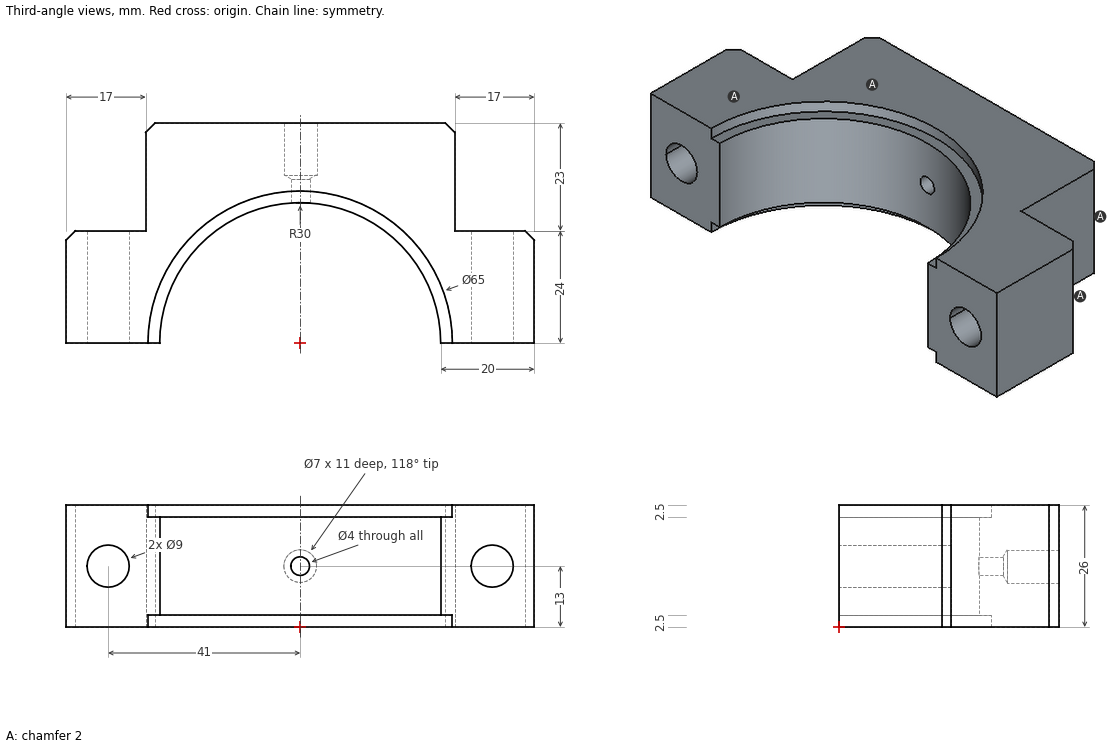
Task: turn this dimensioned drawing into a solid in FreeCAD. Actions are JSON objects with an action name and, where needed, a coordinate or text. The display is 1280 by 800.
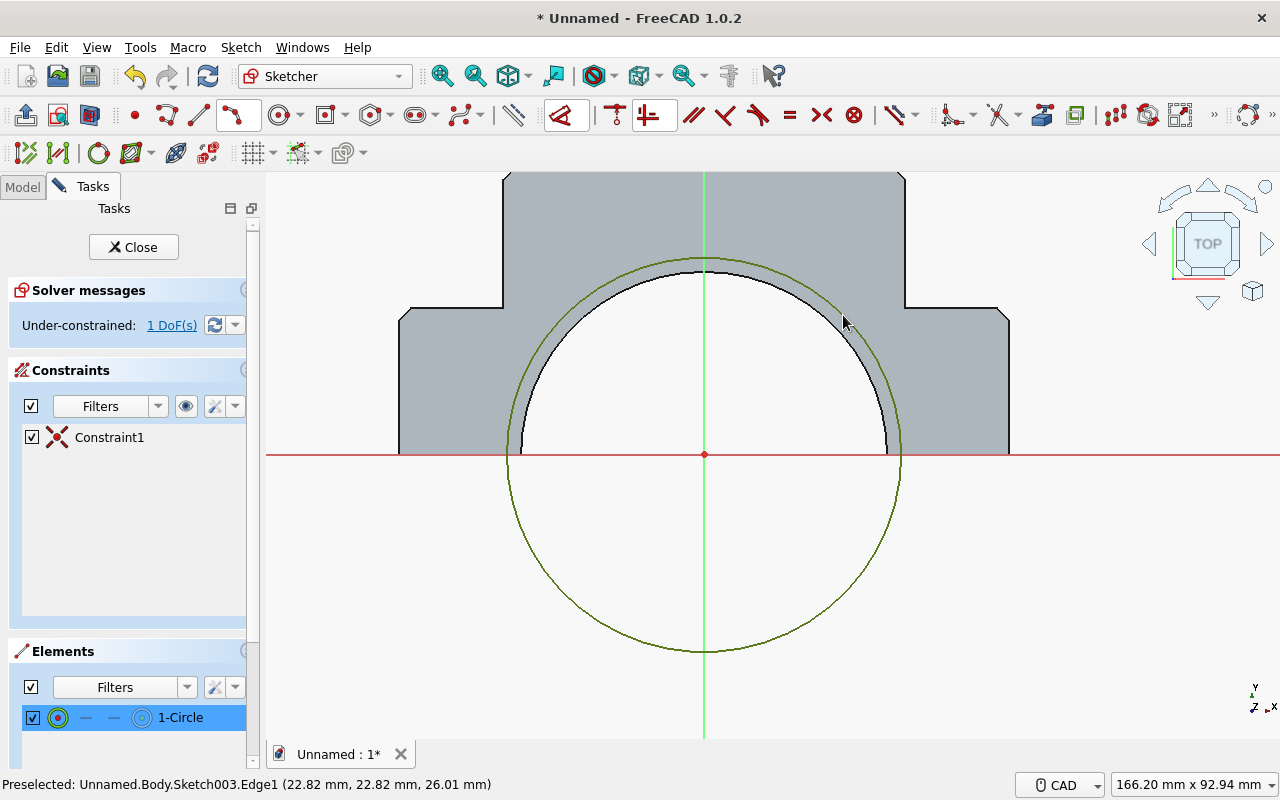
{"action": "key", "text": "k o"}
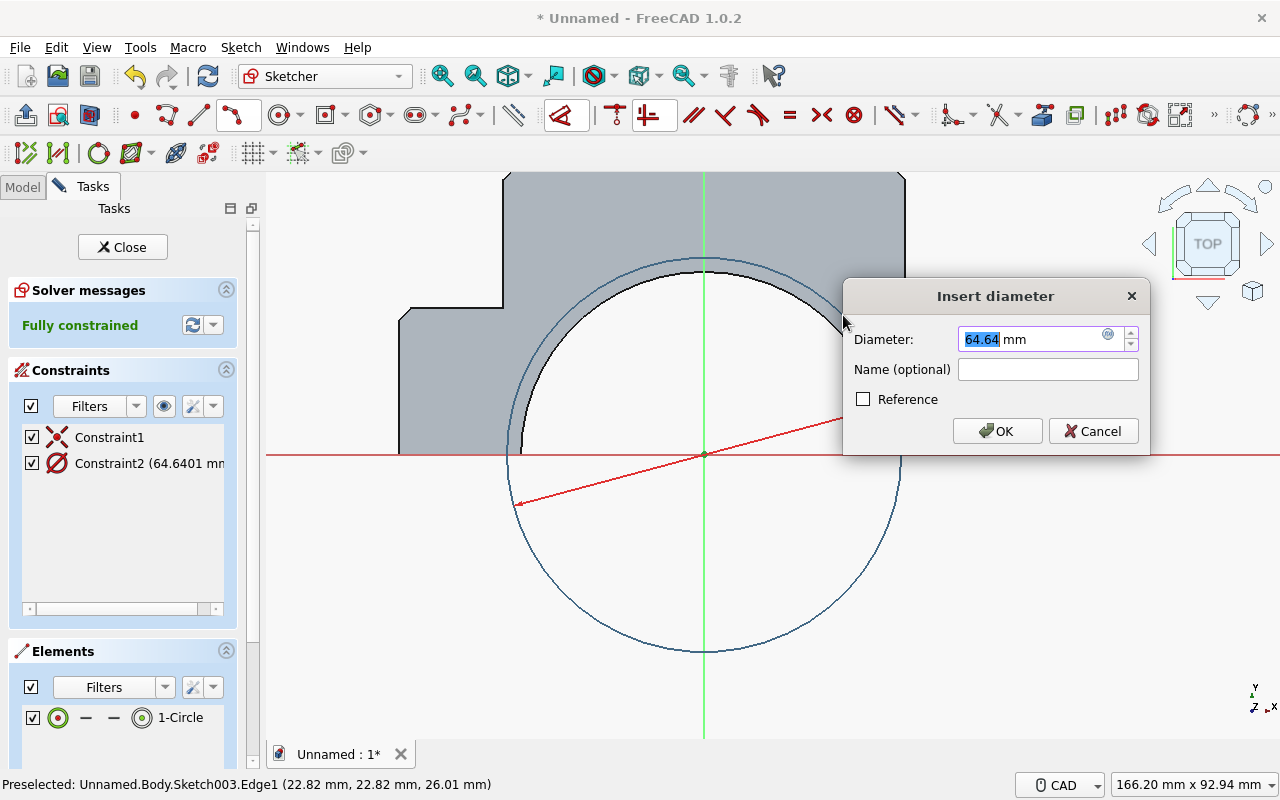
{"action": "type", "text": "65"}
{"action": "key", "text": "Return"}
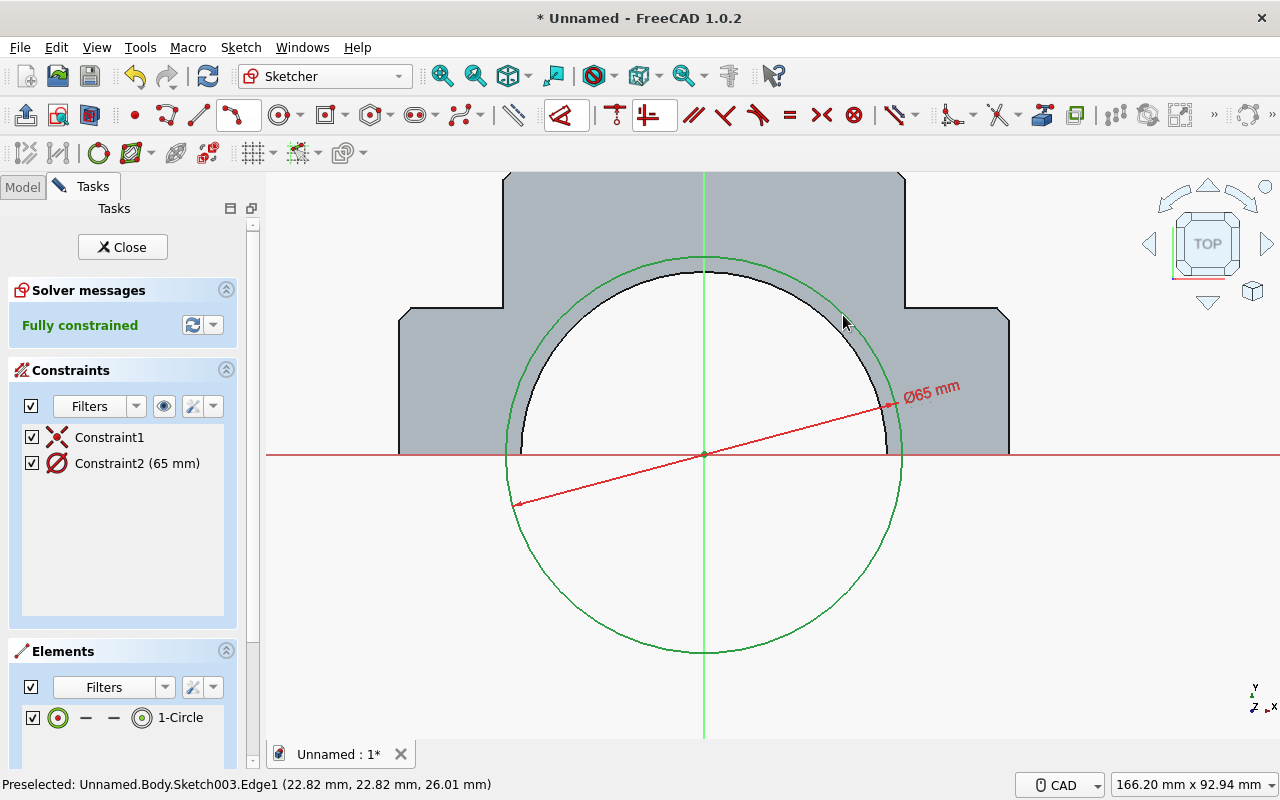
{"action": "left_click", "coordinate": [123, 247]}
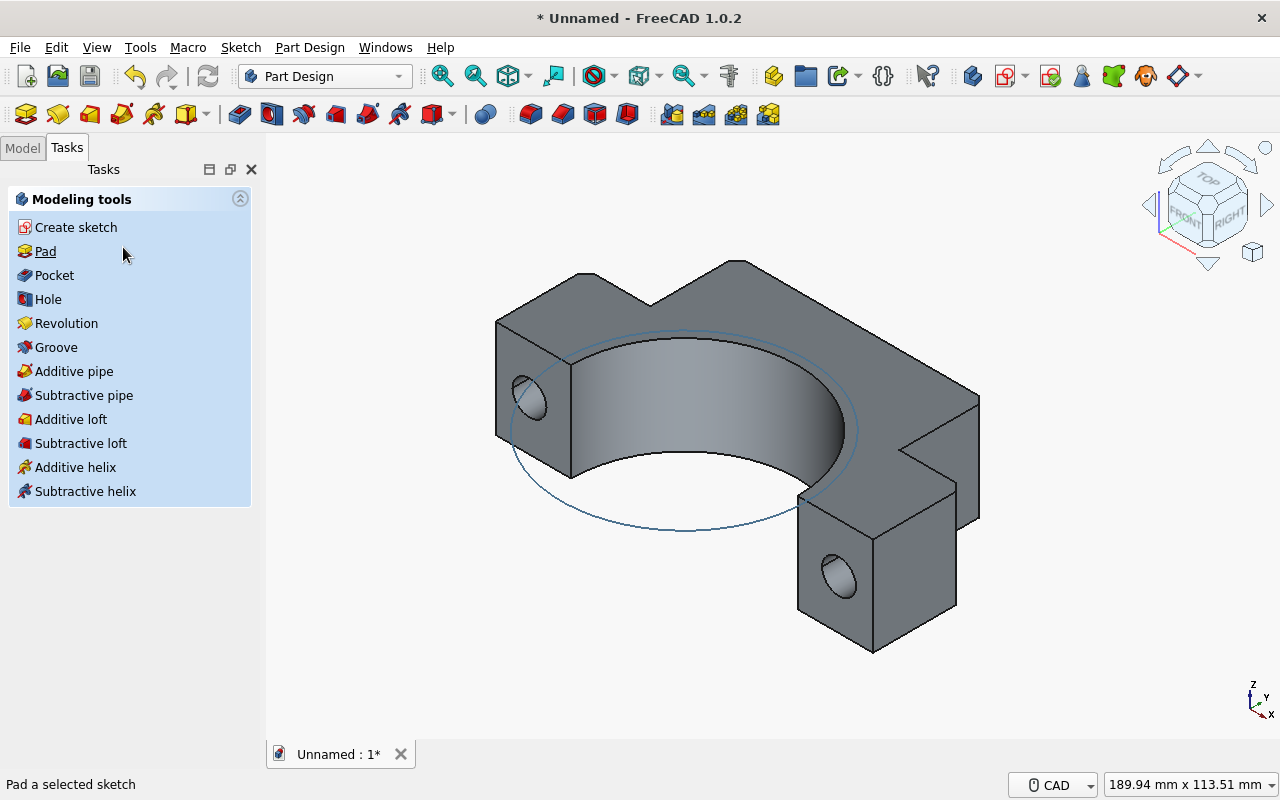
{"action": "left_click", "coordinate": [240, 114]}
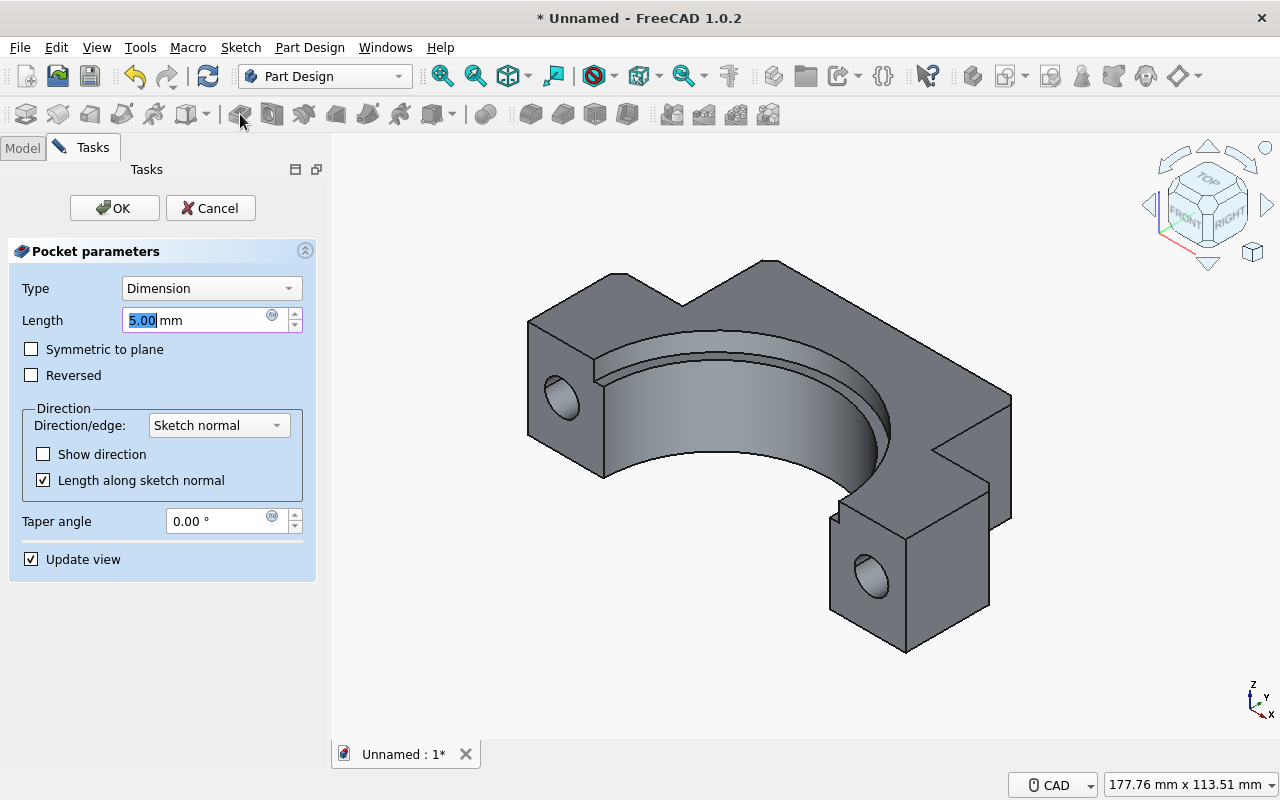
{"action": "type", "text": "2.5"}
{"action": "key", "text": "Tab"}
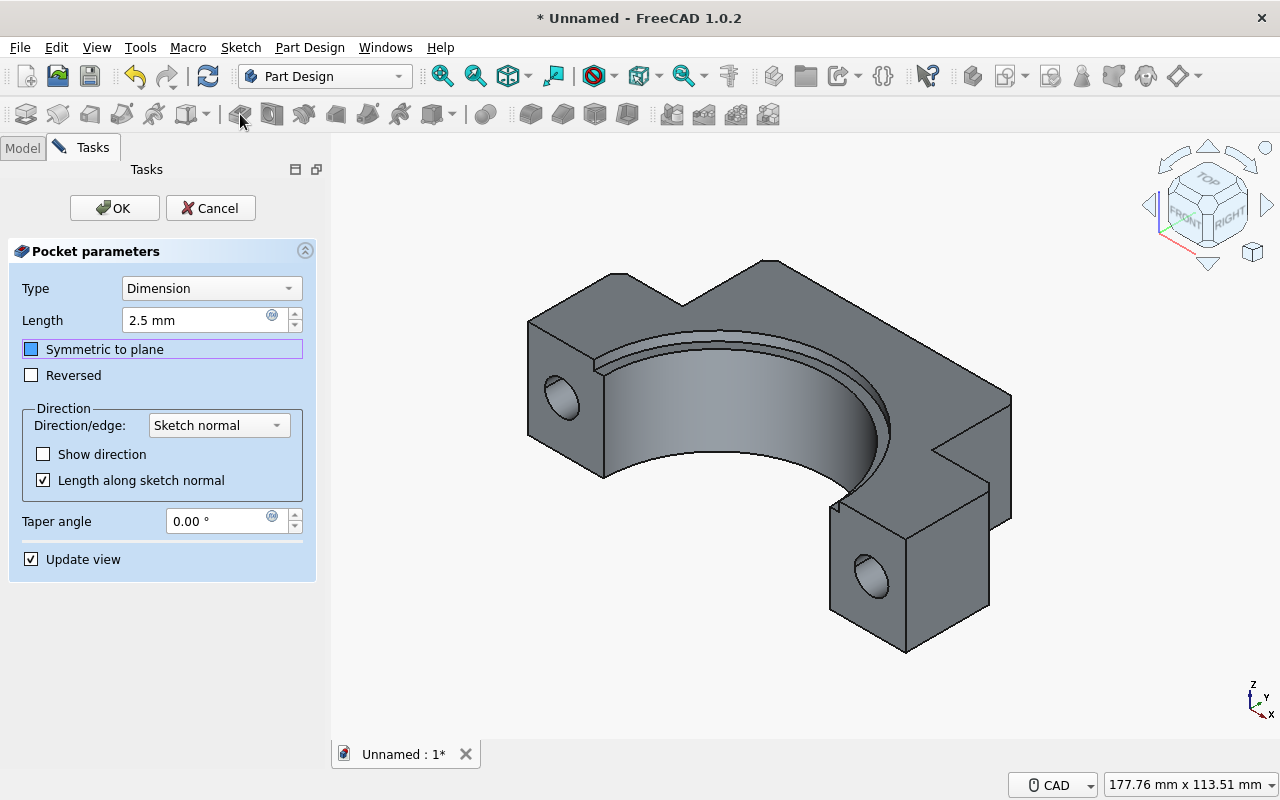
{"action": "left_click", "coordinate": [115, 208]}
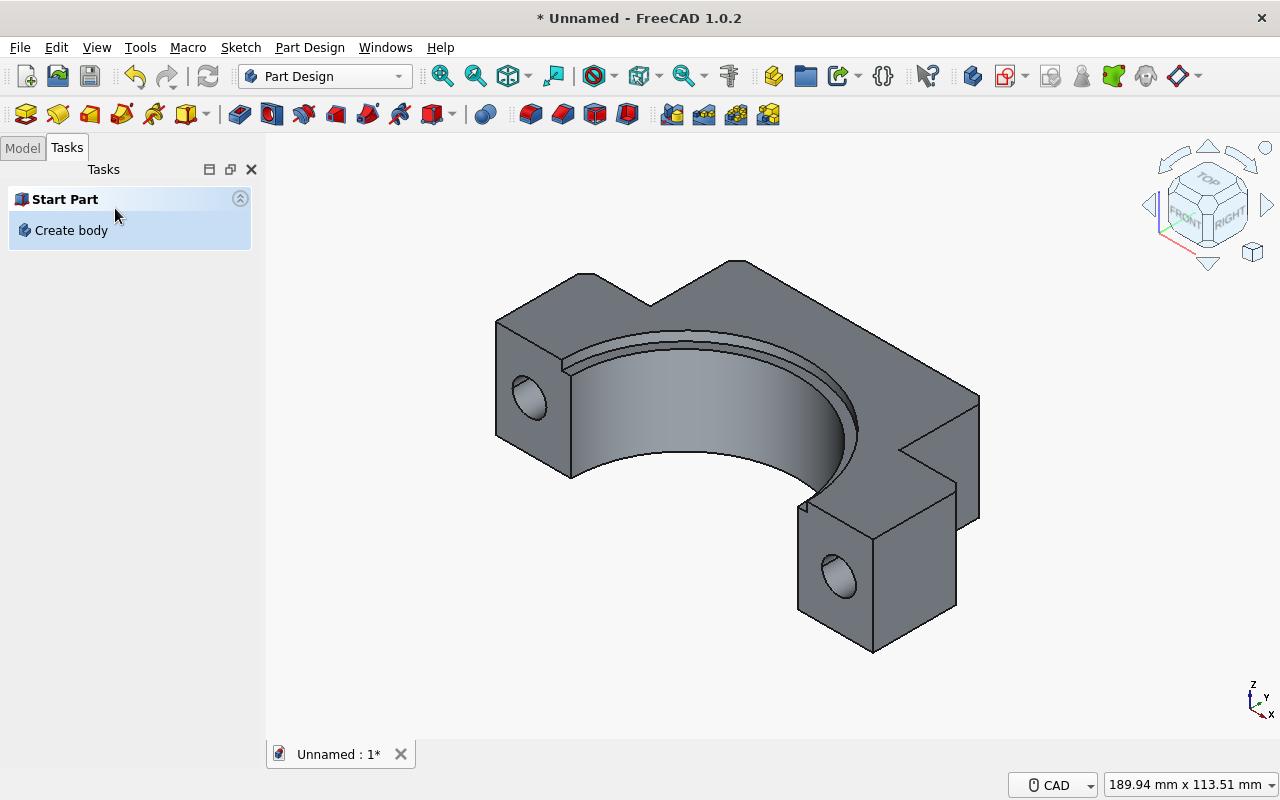
{"action": "left_click", "coordinate": [23, 147]}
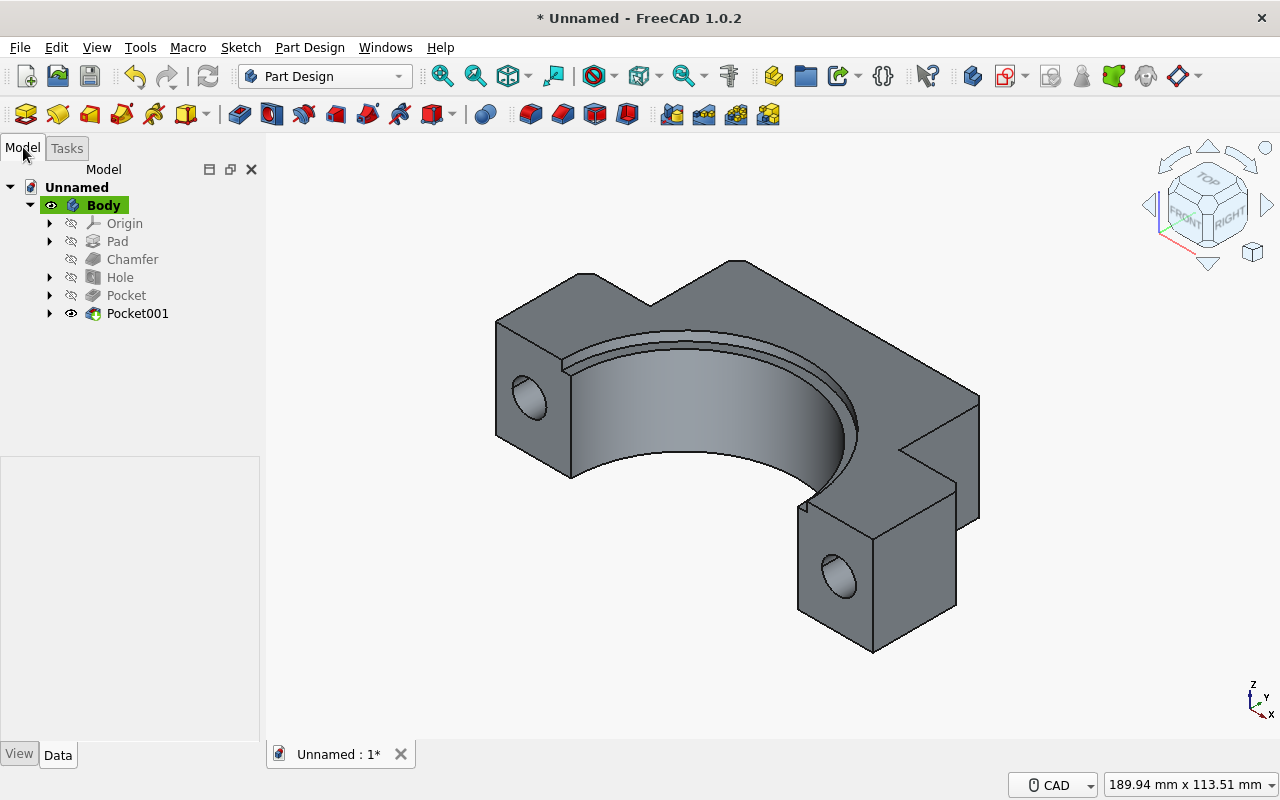
{"action": "left_click", "coordinate": [50, 223]}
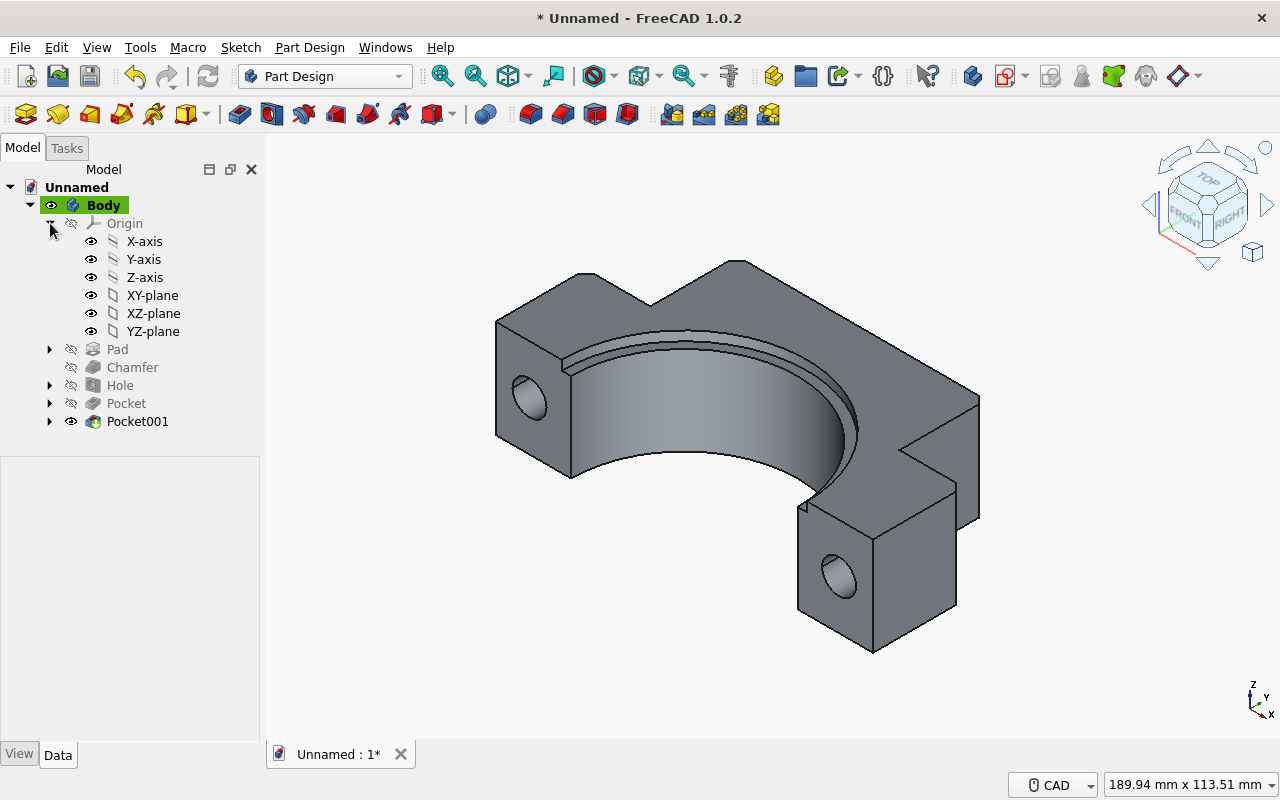
{"action": "left_click", "coordinate": [136, 295]}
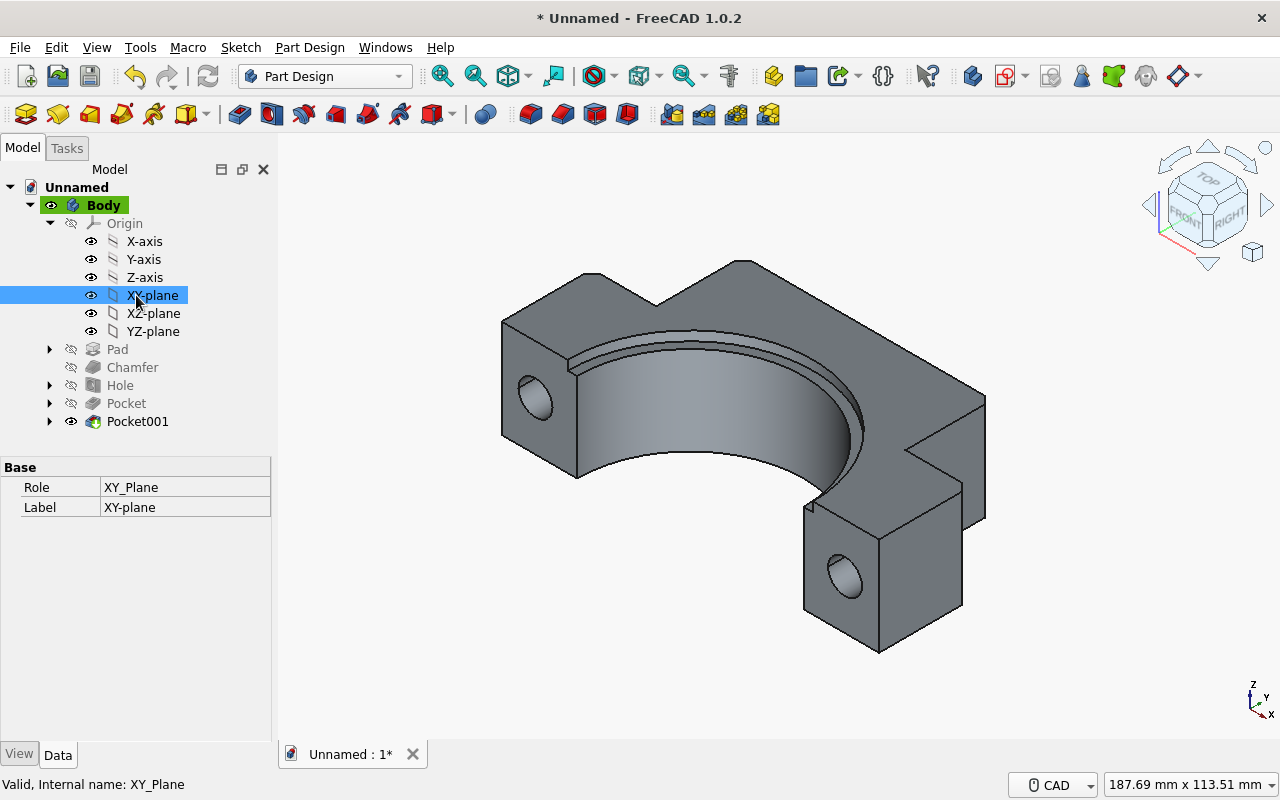
{"action": "left_click", "coordinate": [1178, 76]}